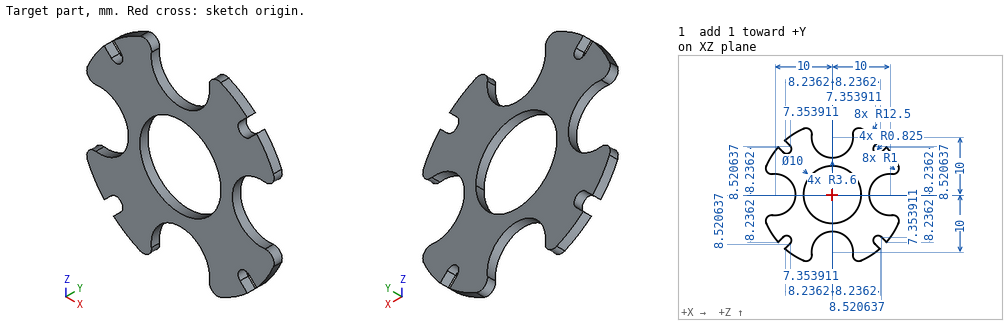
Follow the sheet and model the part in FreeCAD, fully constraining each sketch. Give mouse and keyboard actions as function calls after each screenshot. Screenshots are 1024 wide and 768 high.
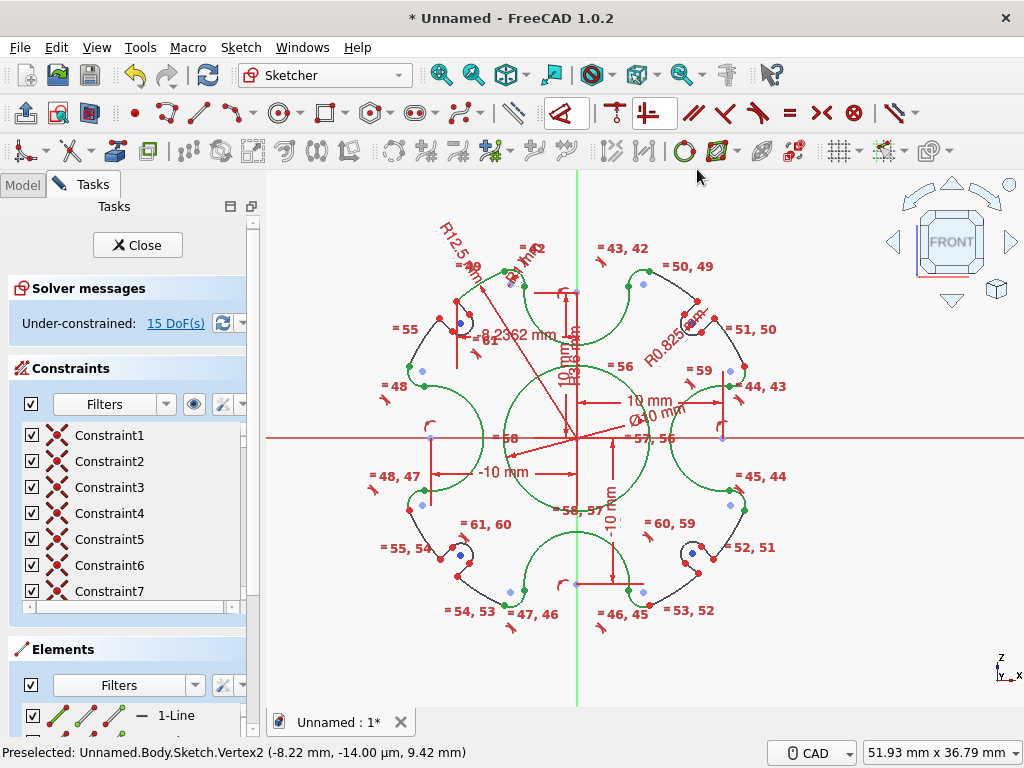
click(698, 302)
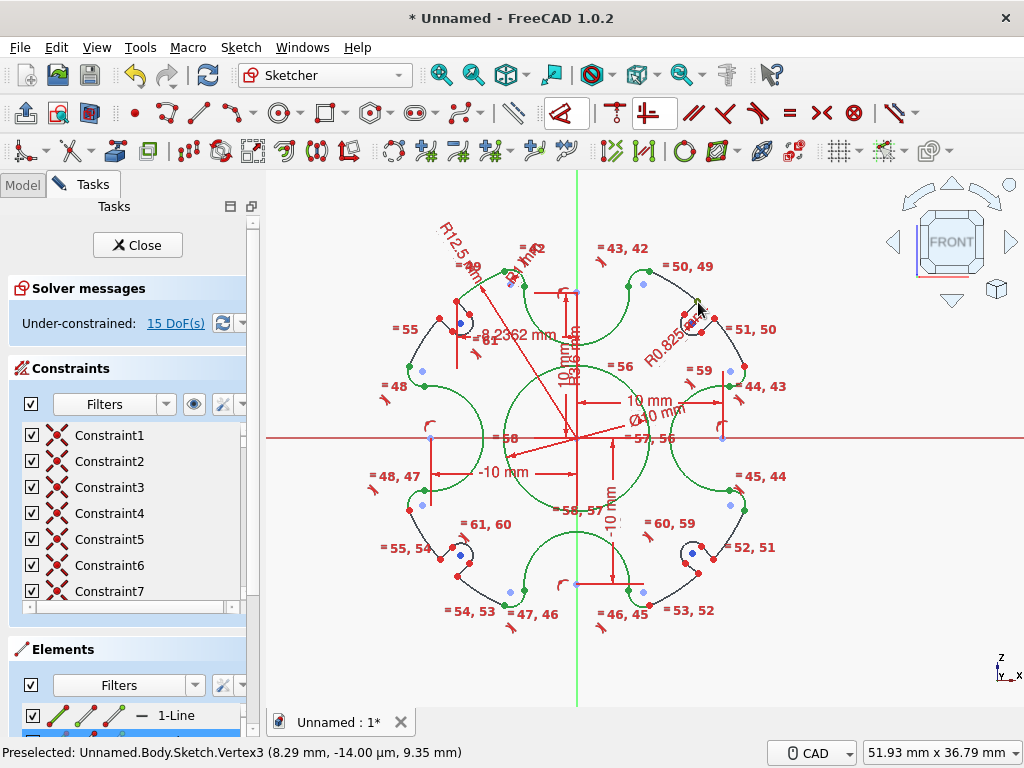
click(584, 114)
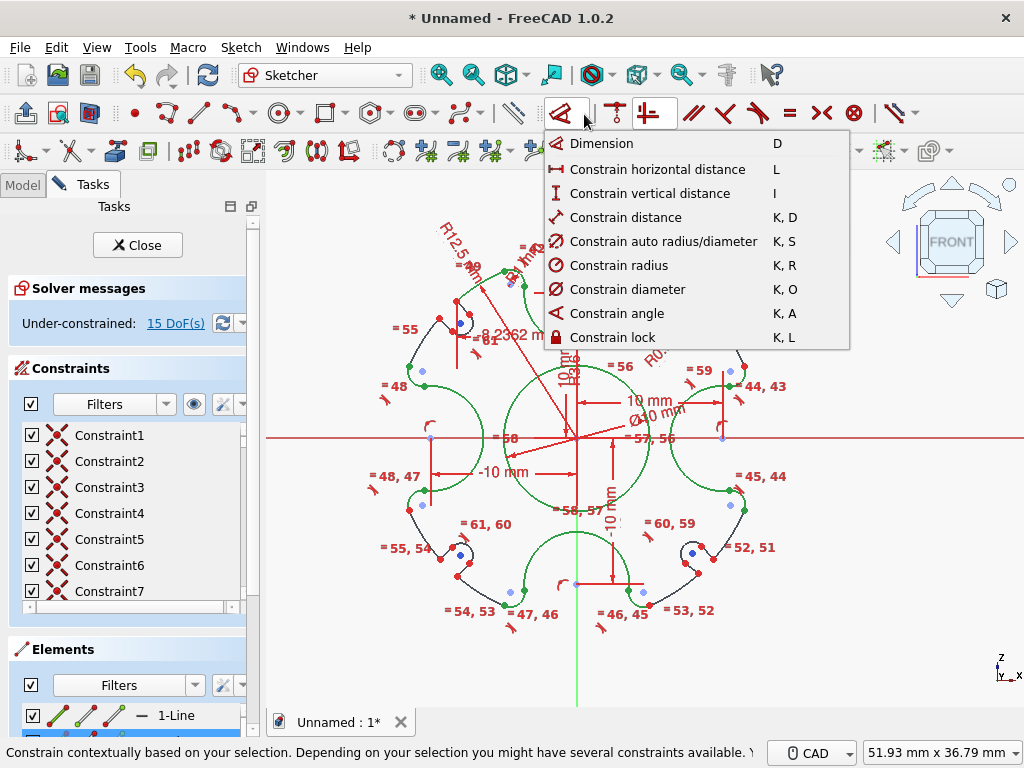
click(697, 169)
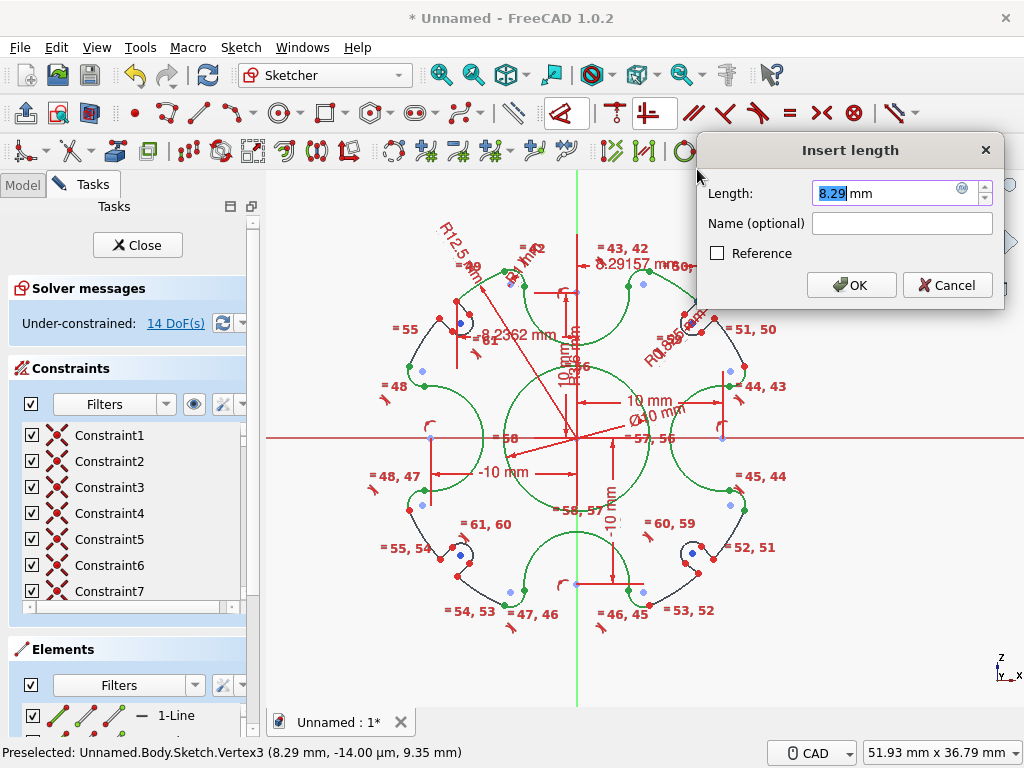
text(8.2362)
key(Return)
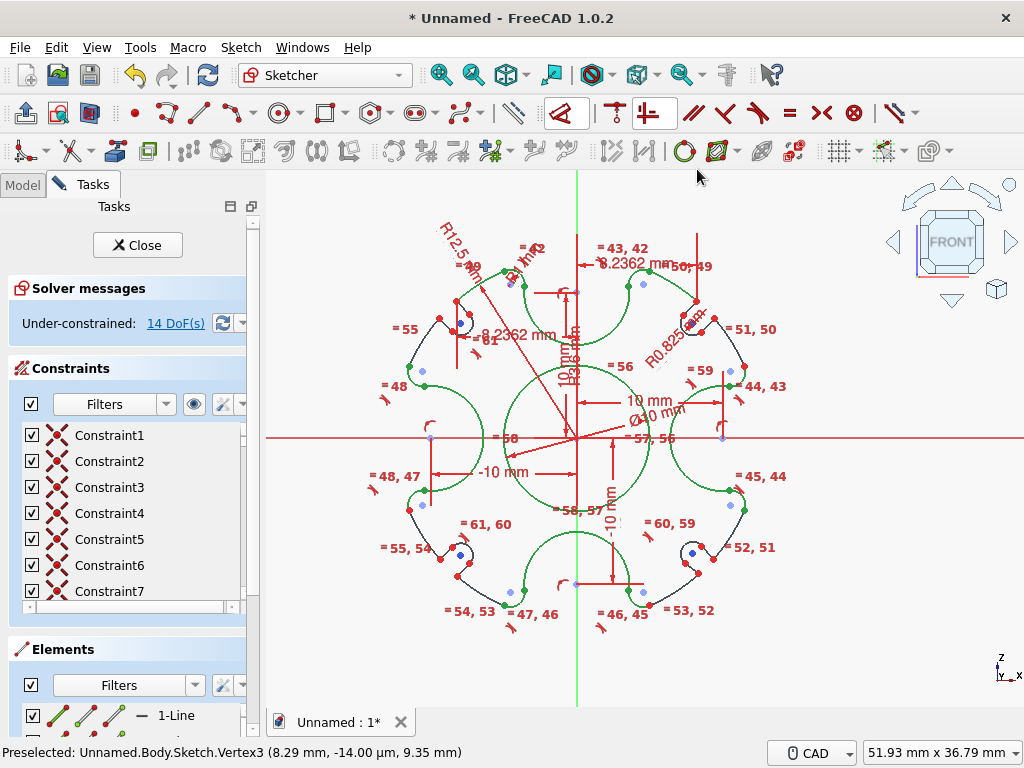
click(715, 319)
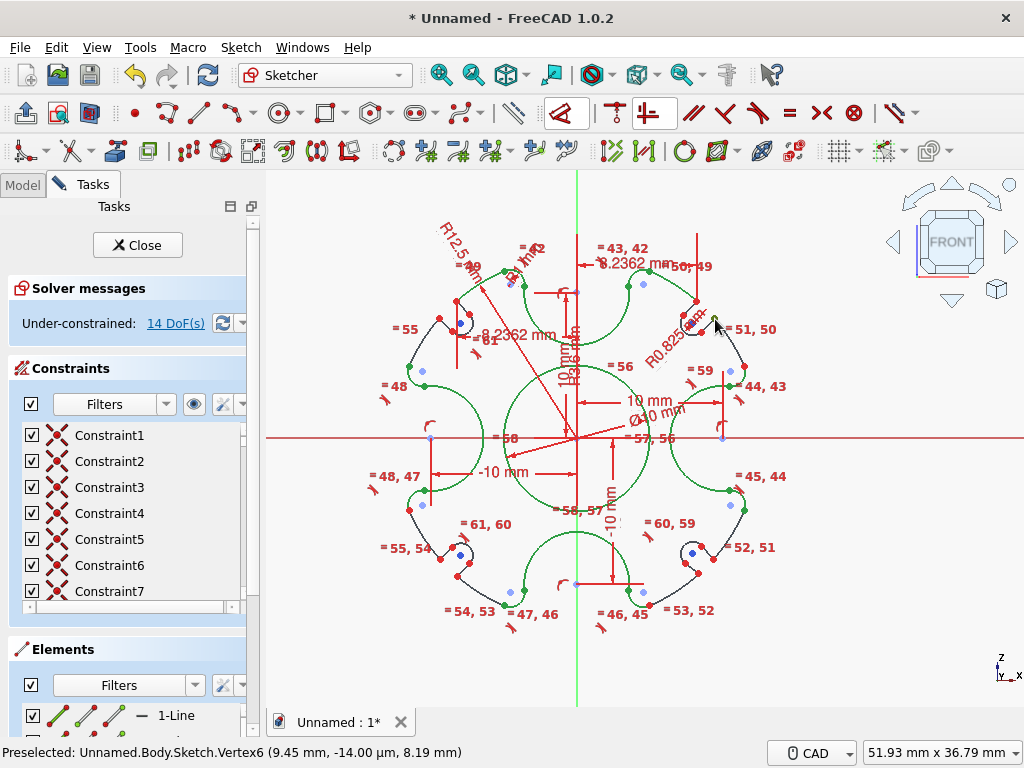
click(584, 114)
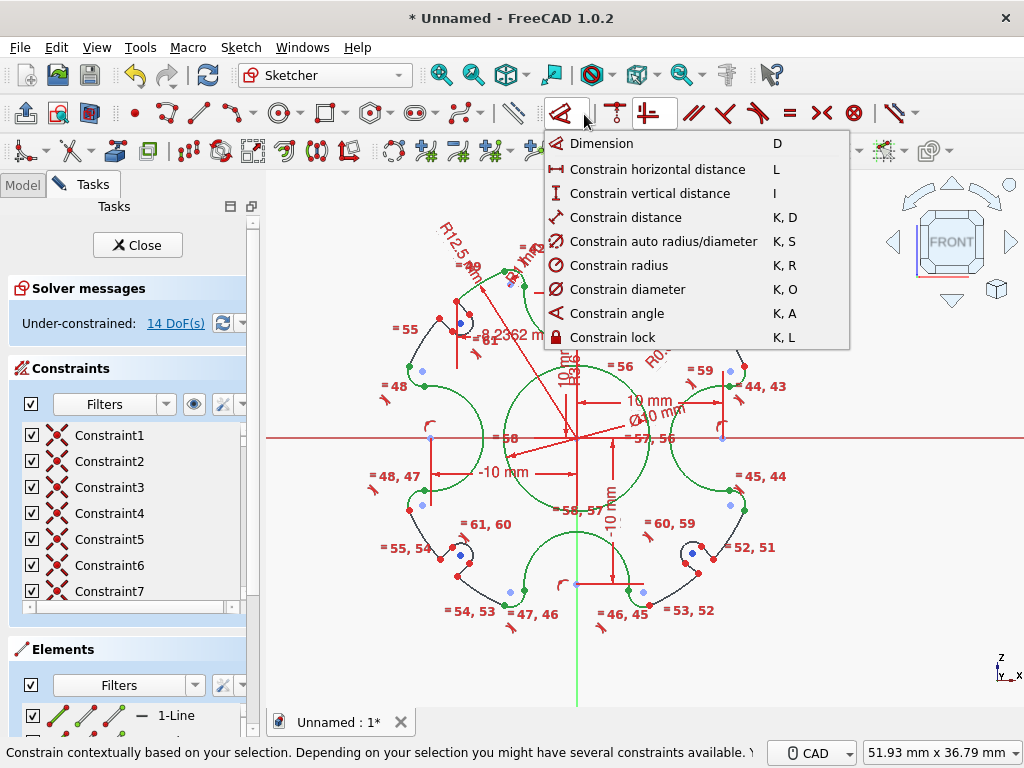
click(697, 193)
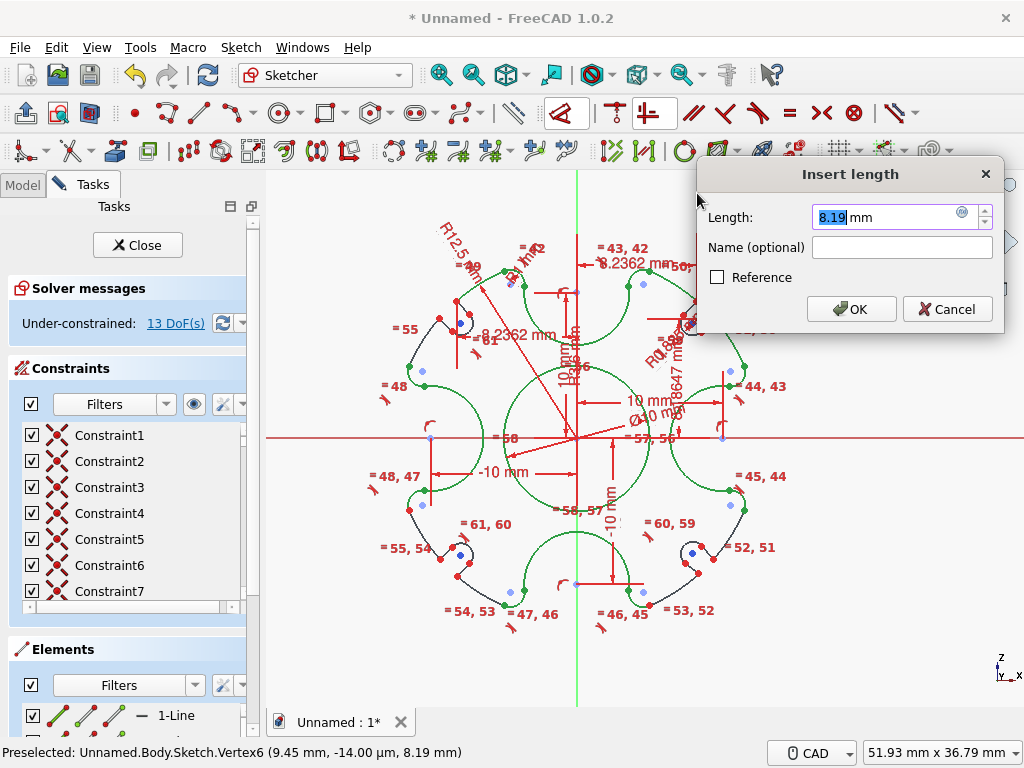
text(8.2362)
key(Return)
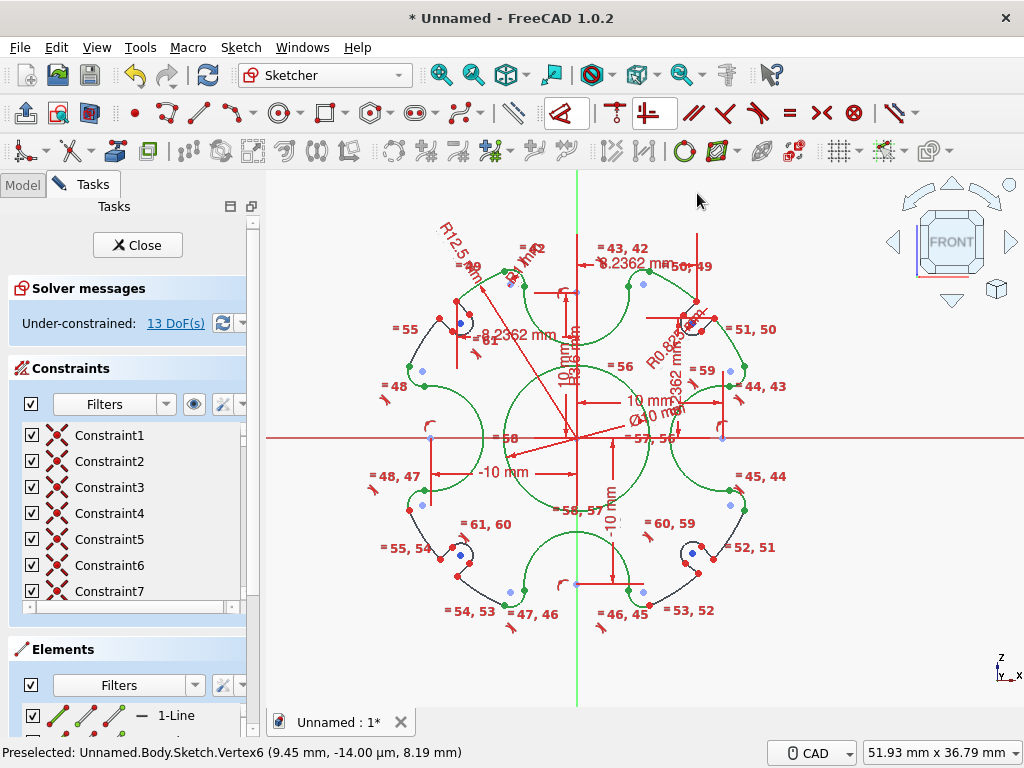
click(713, 560)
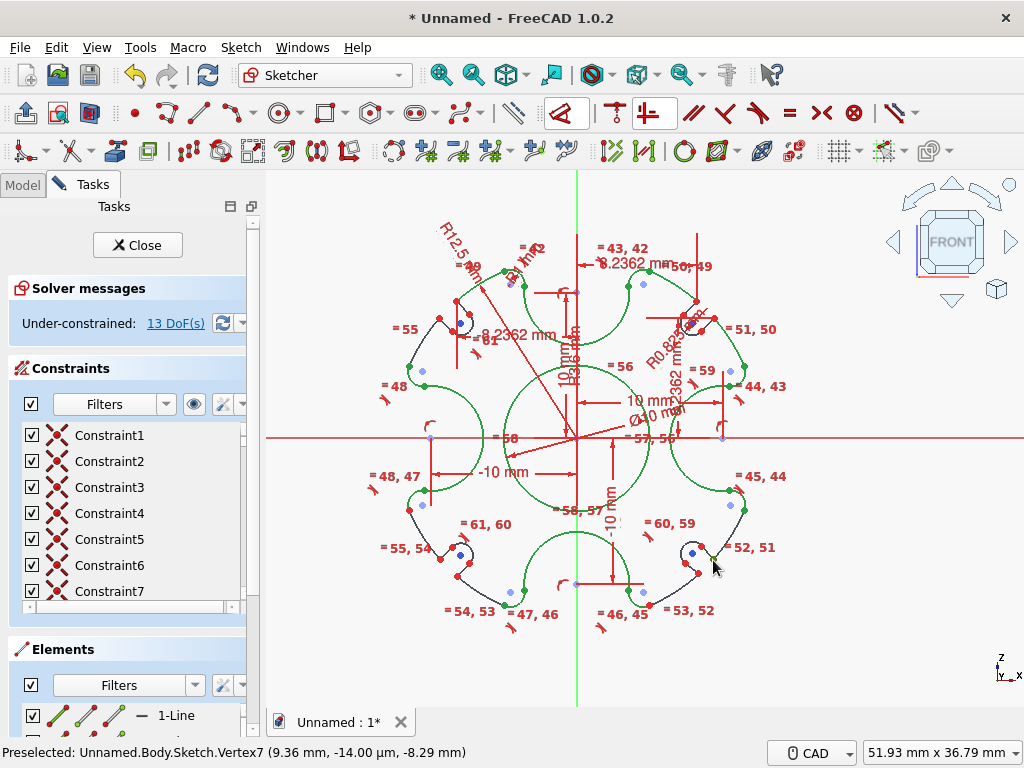
key(i)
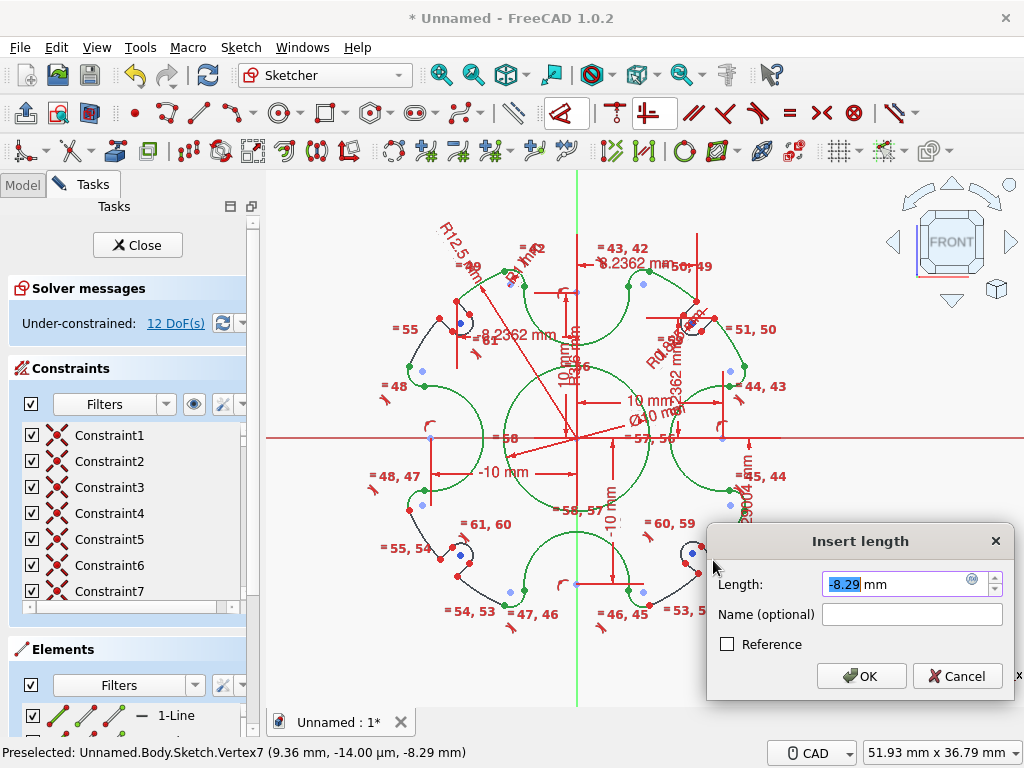
text(-8.2362)
key(Return)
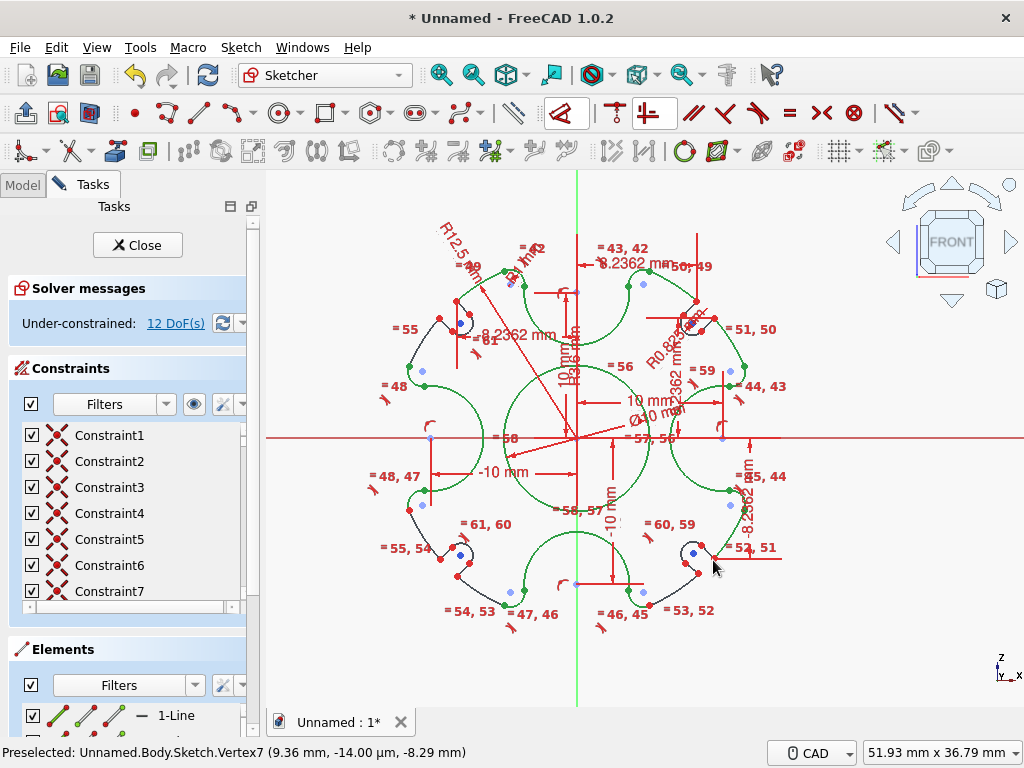
click(699, 574)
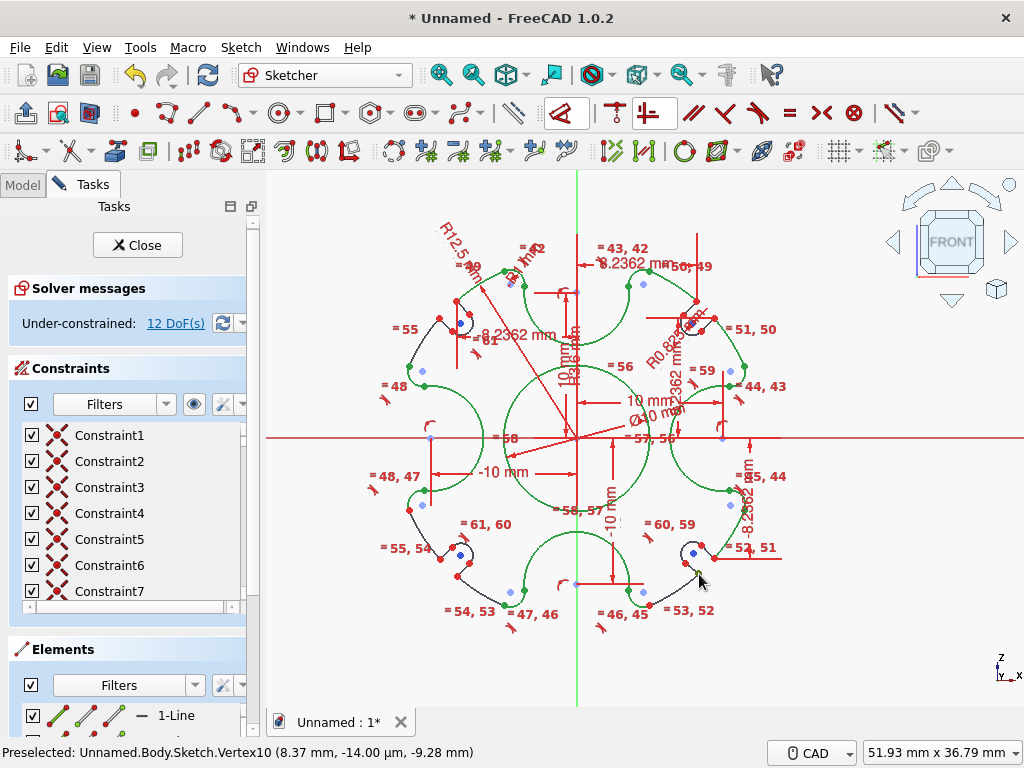
click(584, 114)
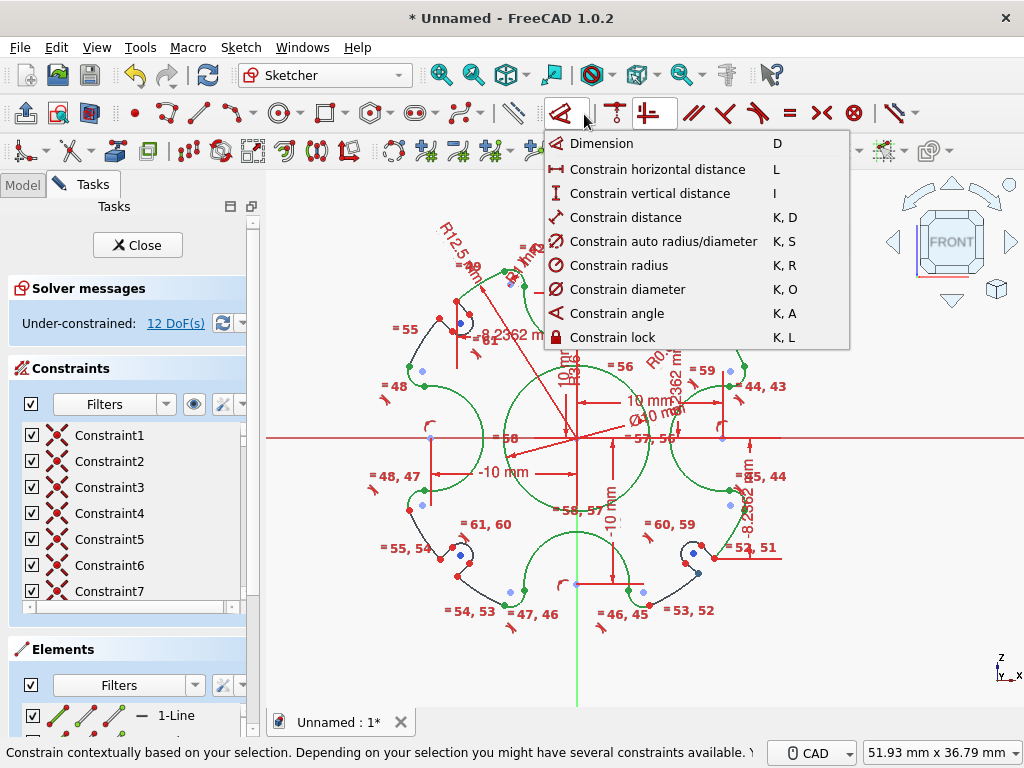
click(697, 169)